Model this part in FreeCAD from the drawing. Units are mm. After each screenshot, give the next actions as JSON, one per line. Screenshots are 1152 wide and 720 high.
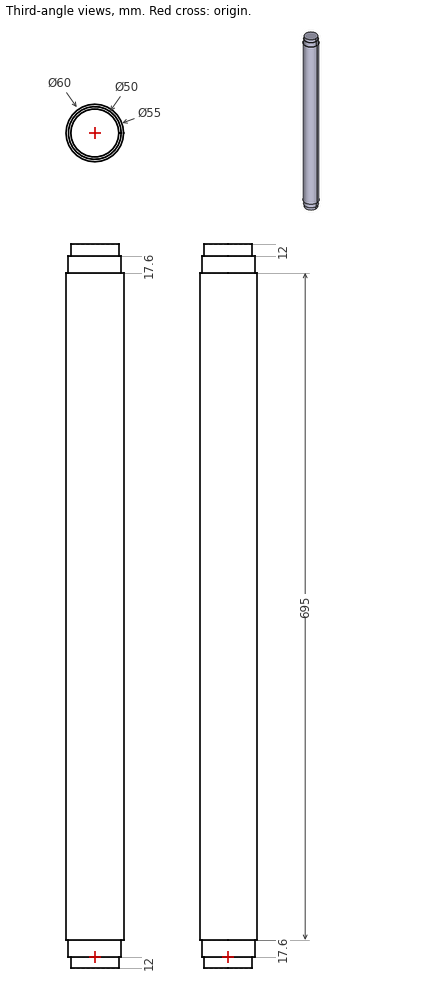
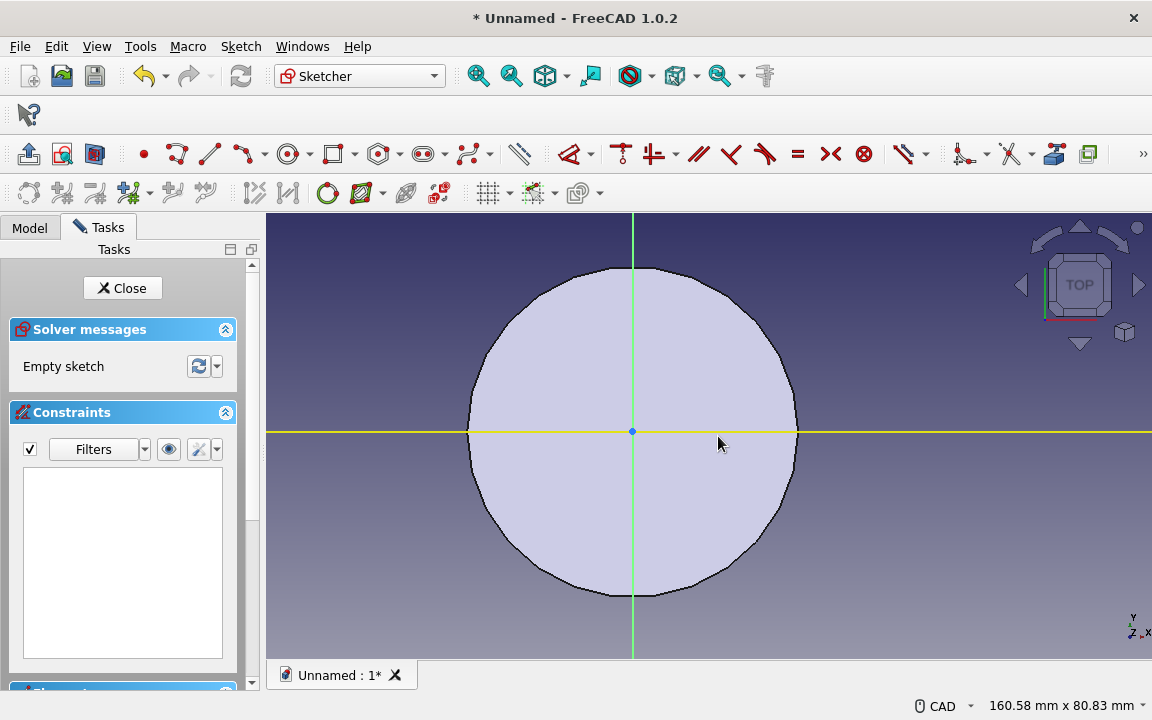
{"action": "left_click", "coordinate": [288, 154]}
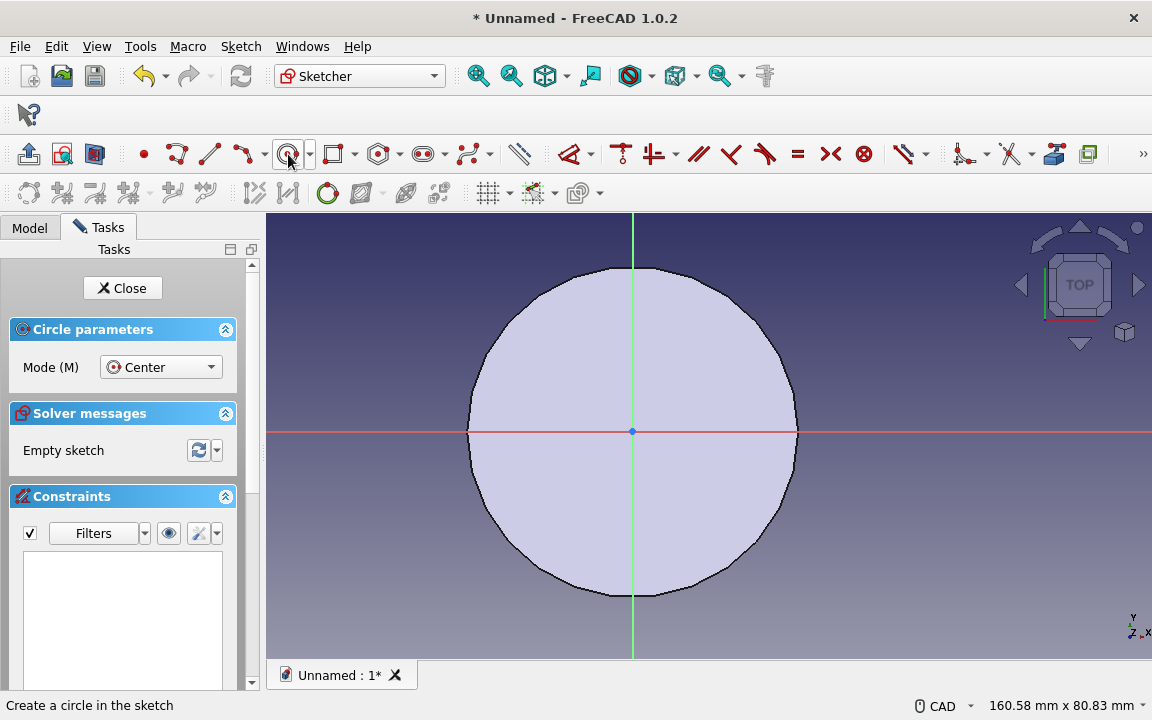
{"action": "left_click", "coordinate": [633, 432]}
{"action": "mouse_move", "coordinate": [740, 325]}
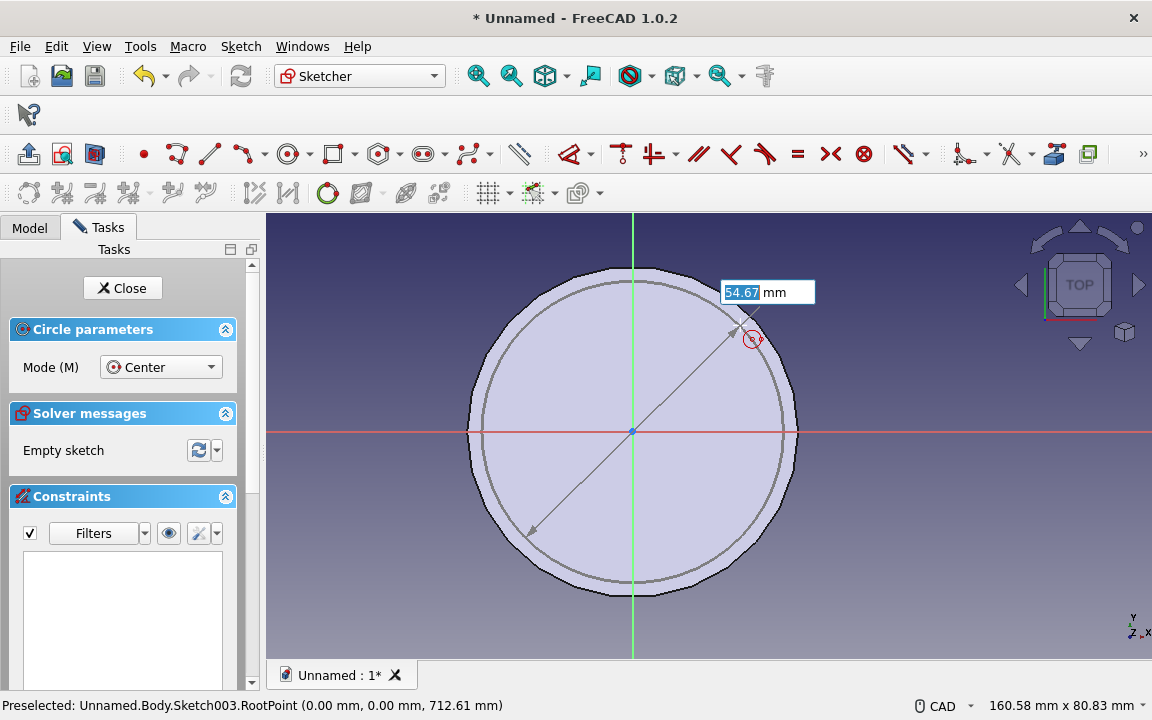
{"action": "type", "text": "55"}
{"action": "key", "text": "Return"}
{"action": "key", "text": "Escape"}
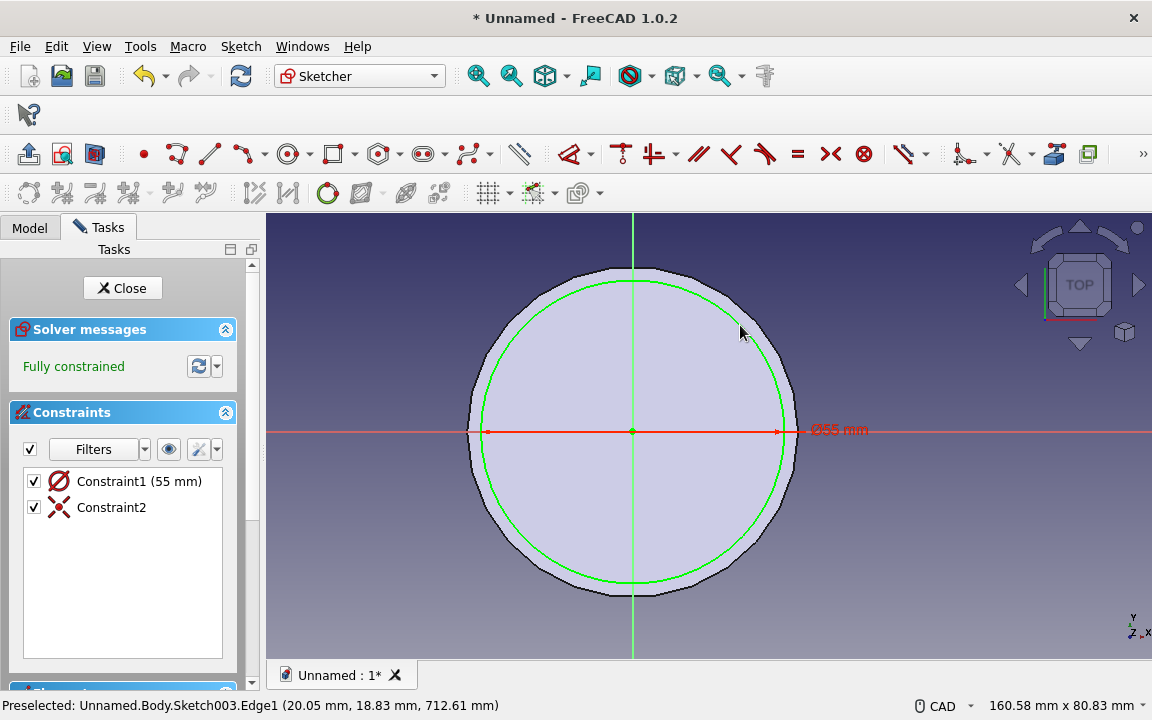
{"action": "left_click", "coordinate": [123, 288]}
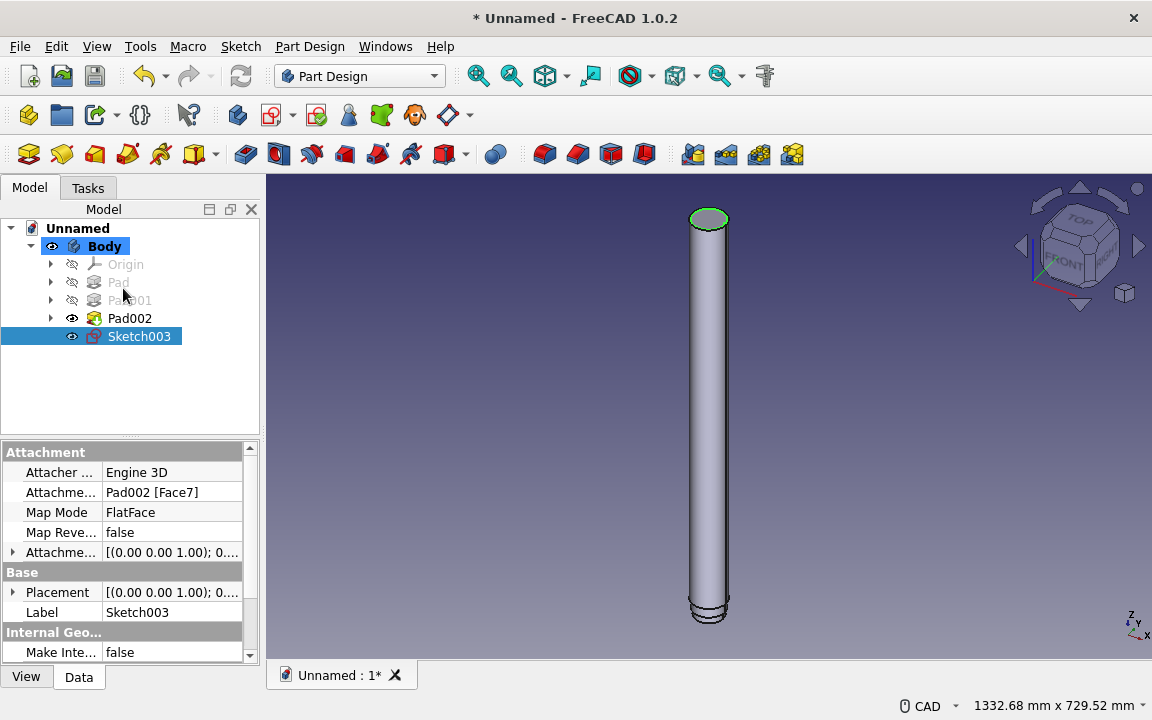
{"action": "left_click", "coordinate": [29, 154]}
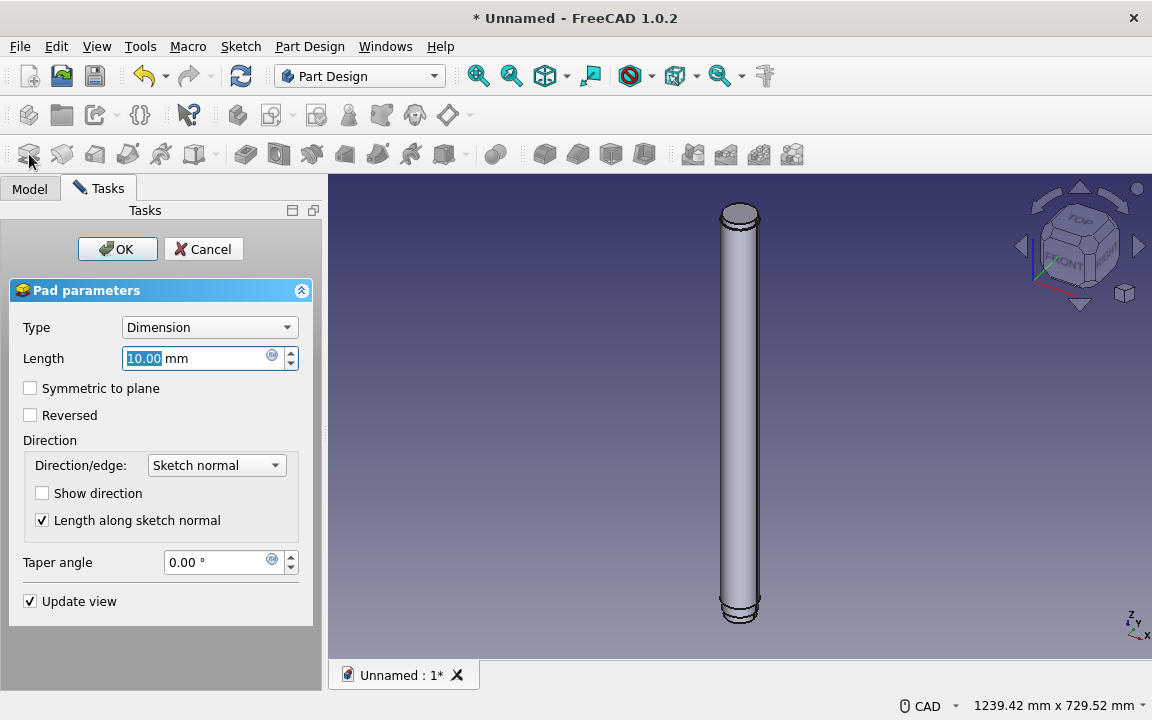
{"action": "type", "text": "17.6"}
{"action": "key", "text": "Tab"}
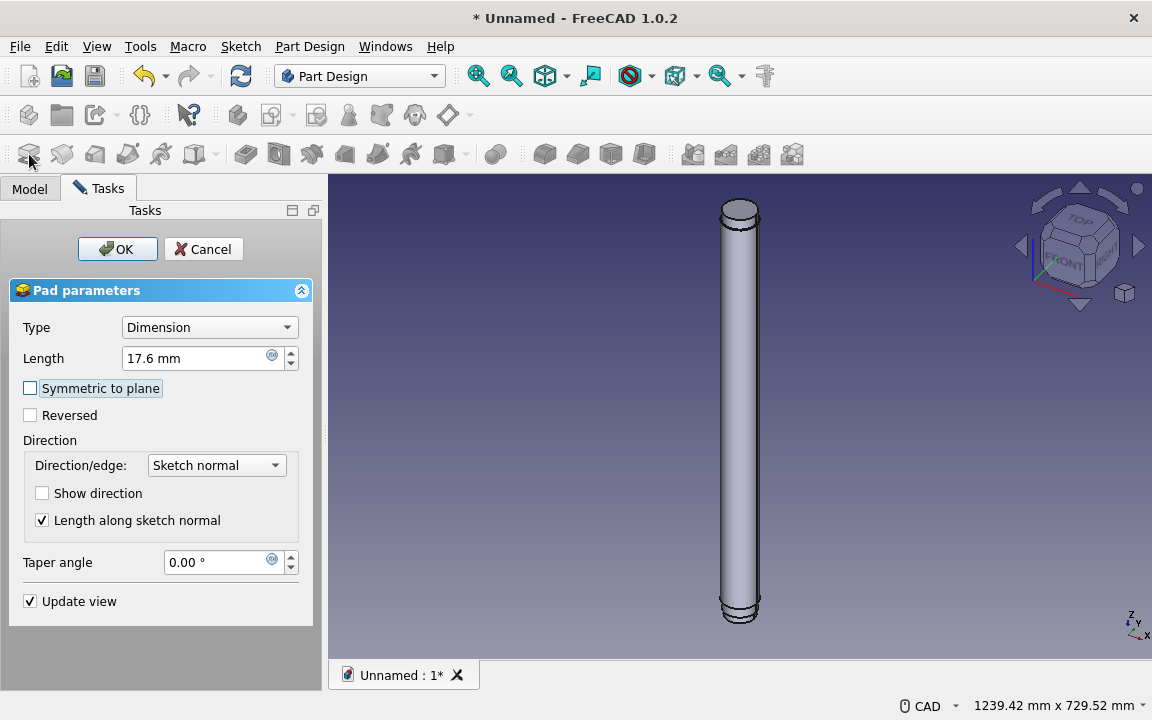
{"action": "left_click", "coordinate": [118, 249]}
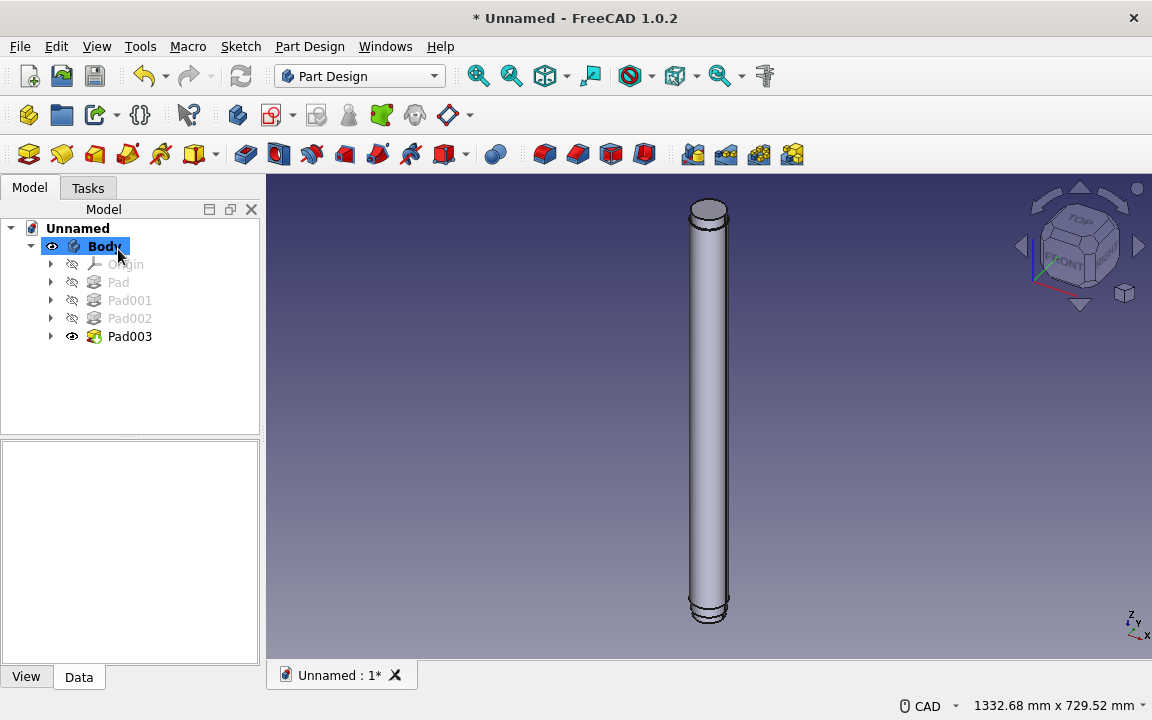
{"action": "left_click", "coordinate": [51, 264]}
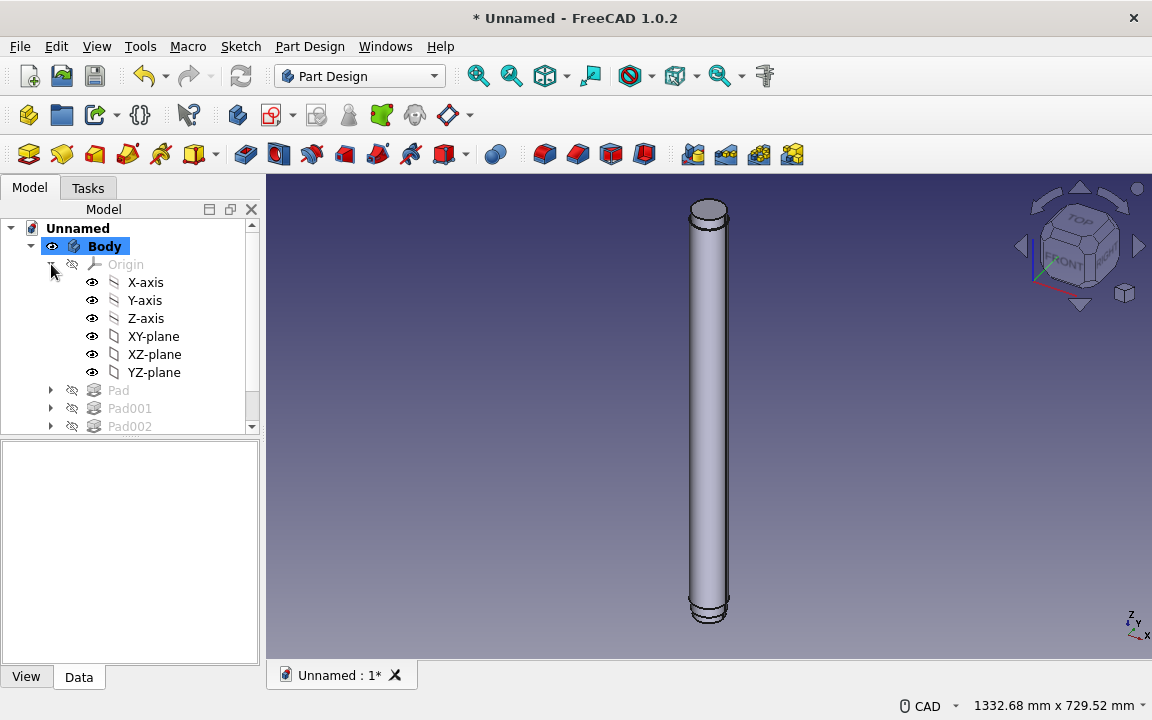
{"action": "left_click", "coordinate": [137, 336]}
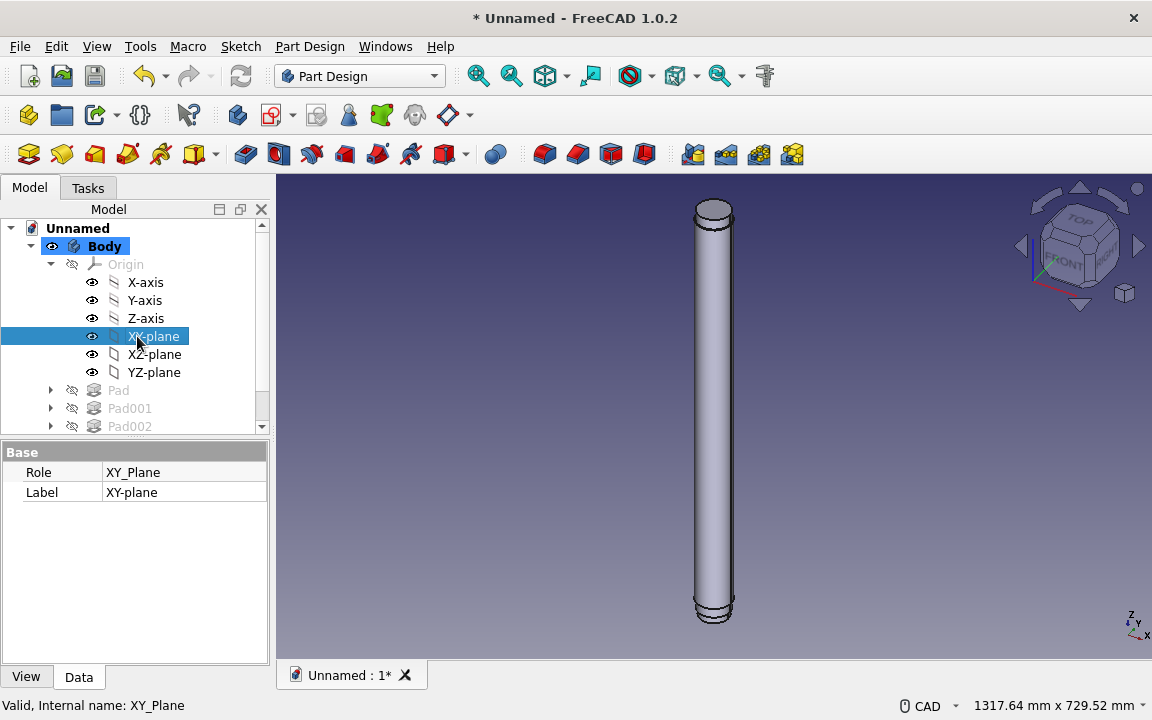
{"action": "left_click", "coordinate": [448, 116]}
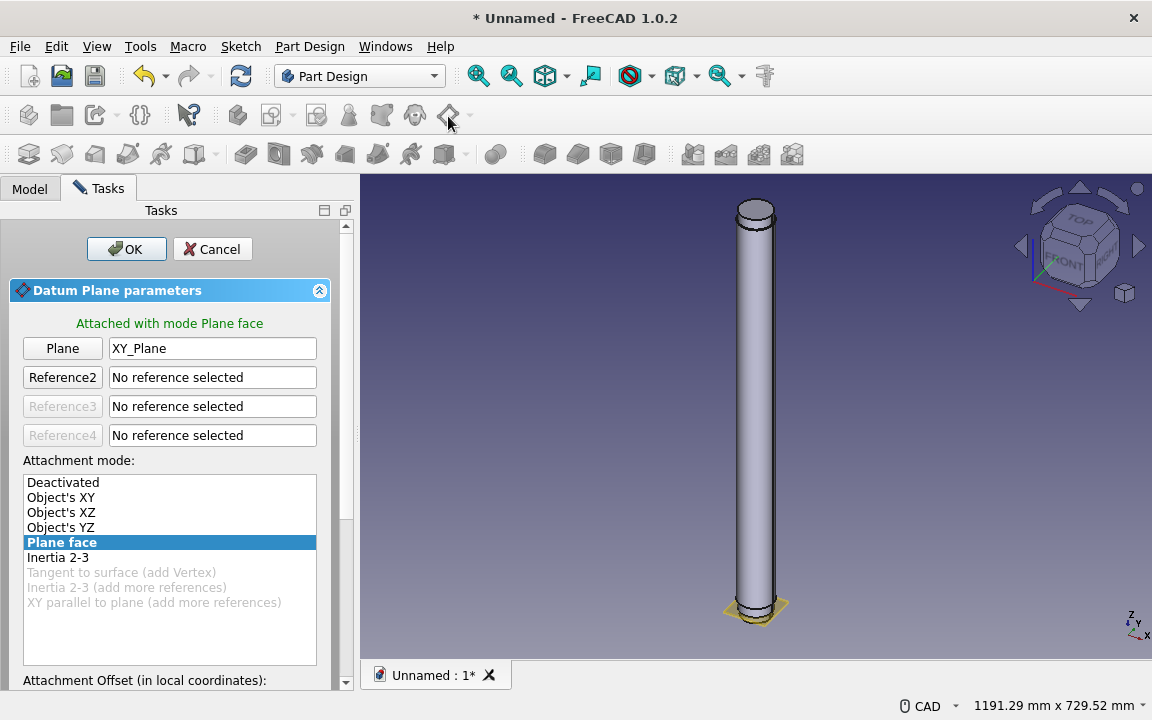
{"action": "scroll", "coordinate": [346, 455], "scroll_direction": "down", "scroll_amount": 3}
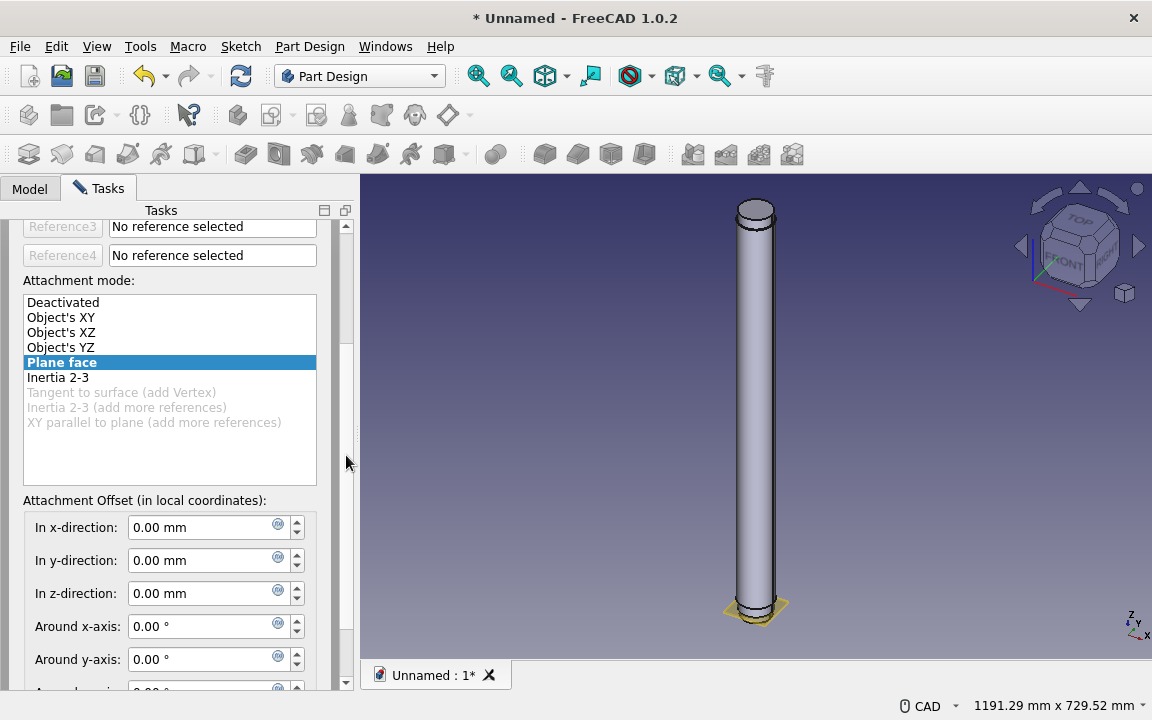
{"action": "triple_click", "coordinate": [210, 594]}